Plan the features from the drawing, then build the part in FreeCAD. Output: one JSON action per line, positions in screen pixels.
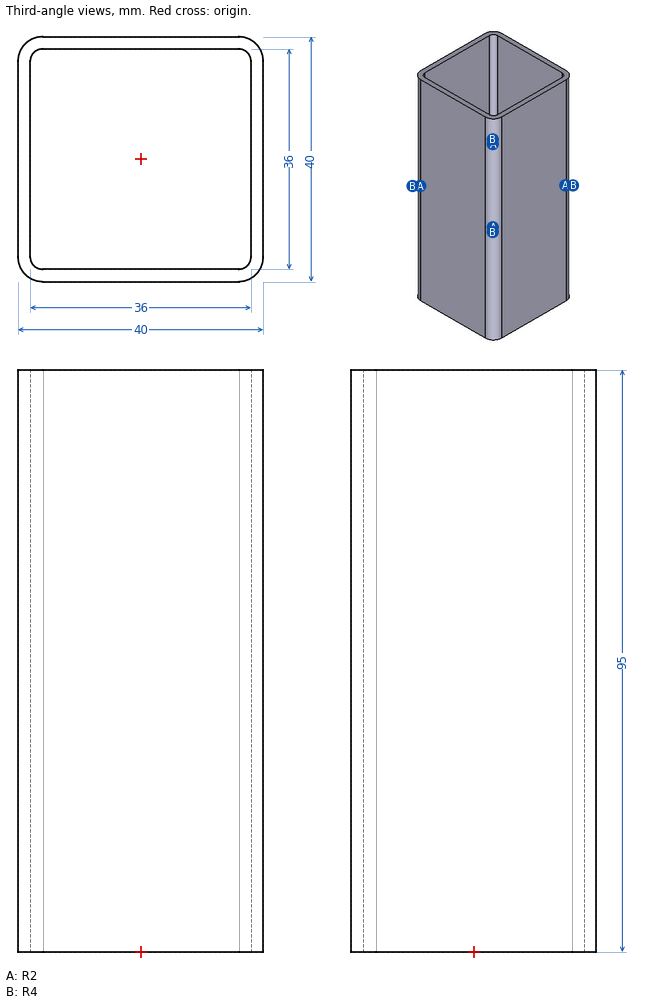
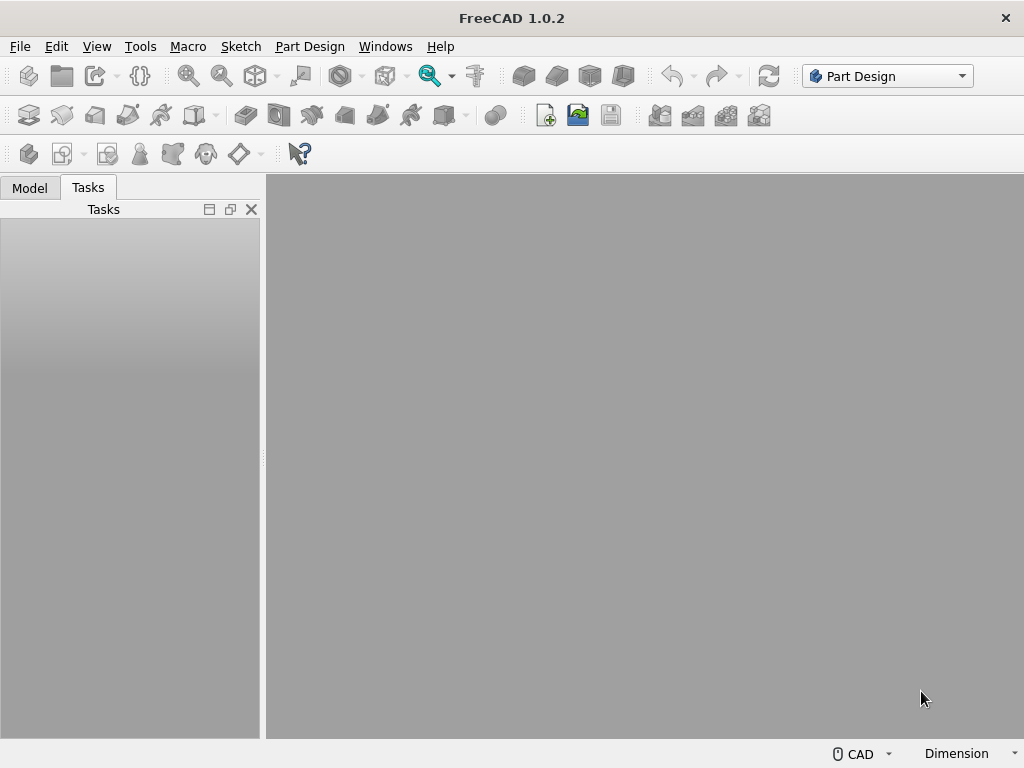
{"action": "left_click", "coordinate": [545, 116]}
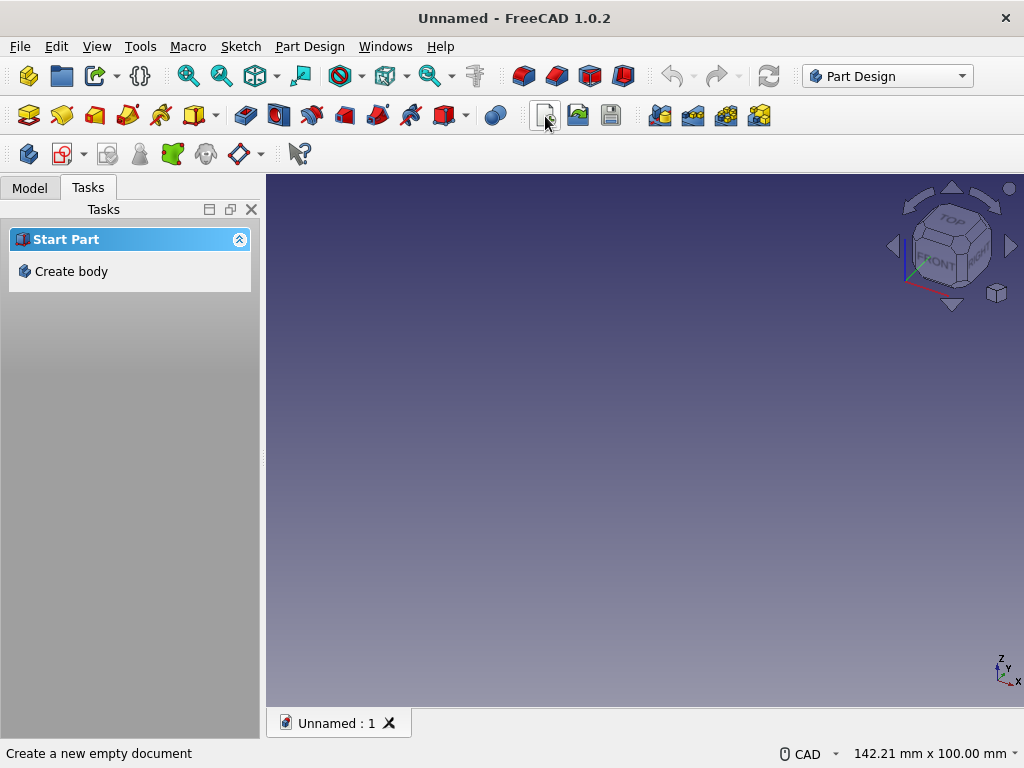
{"action": "left_click", "coordinate": [62, 154]}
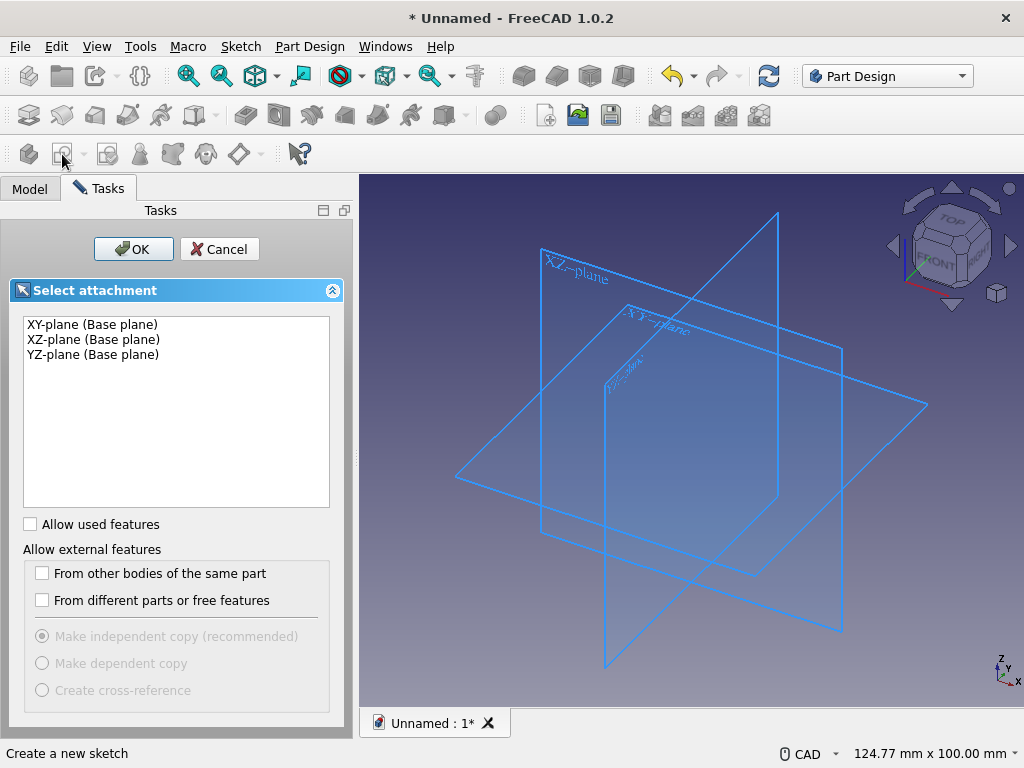
{"action": "left_click", "coordinate": [84, 324]}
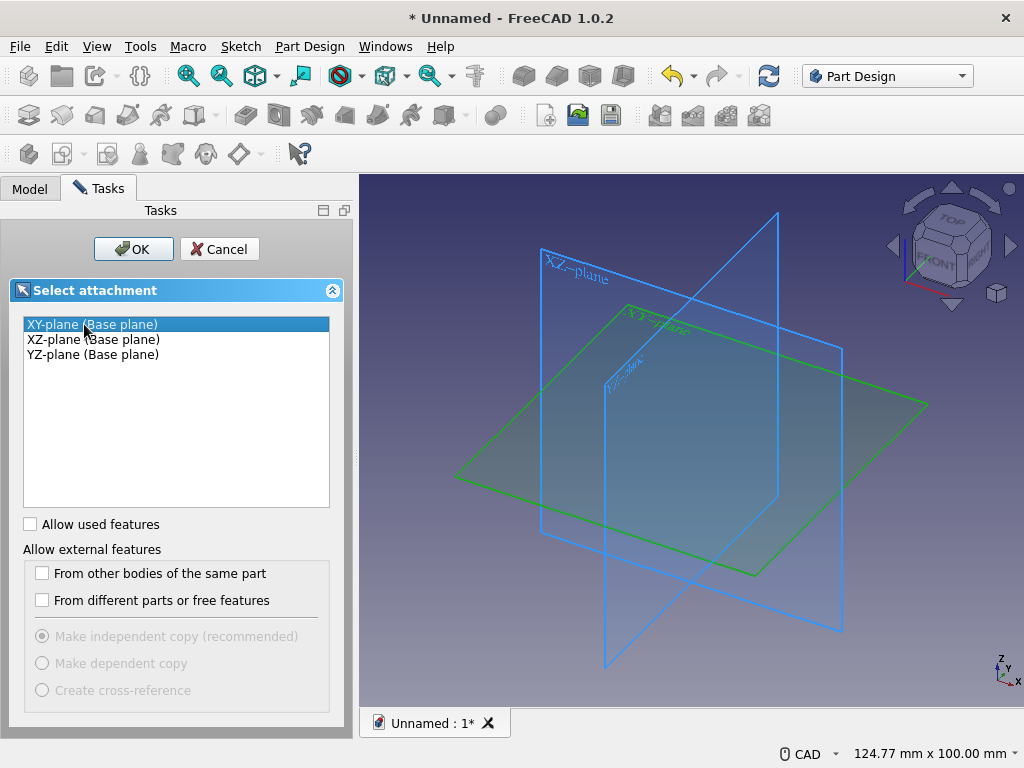
{"action": "left_click", "coordinate": [134, 249]}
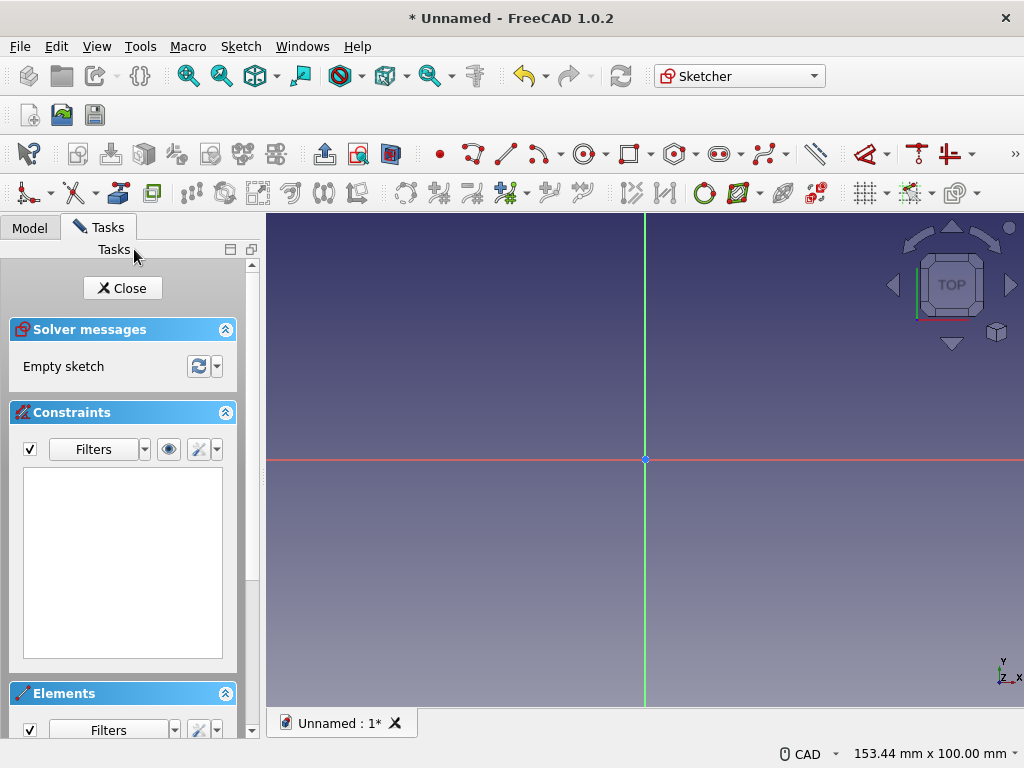
{"action": "scroll", "coordinate": [784, 460], "scroll_direction": "up", "scroll_amount": 2}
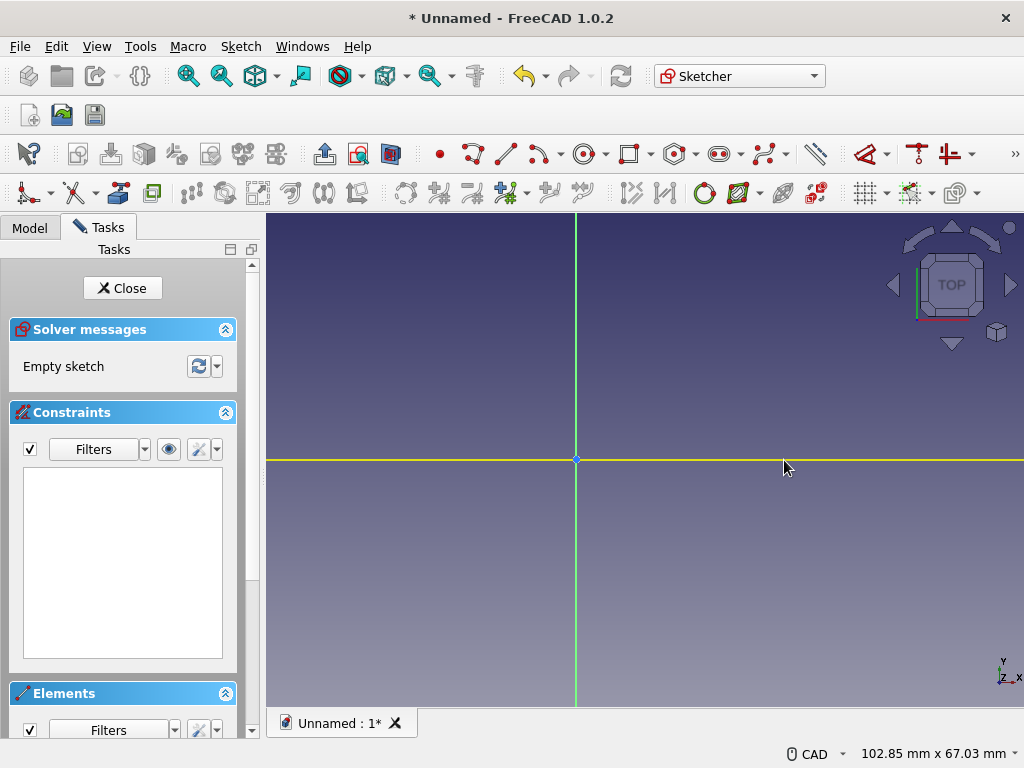
{"action": "key", "text": "g v"}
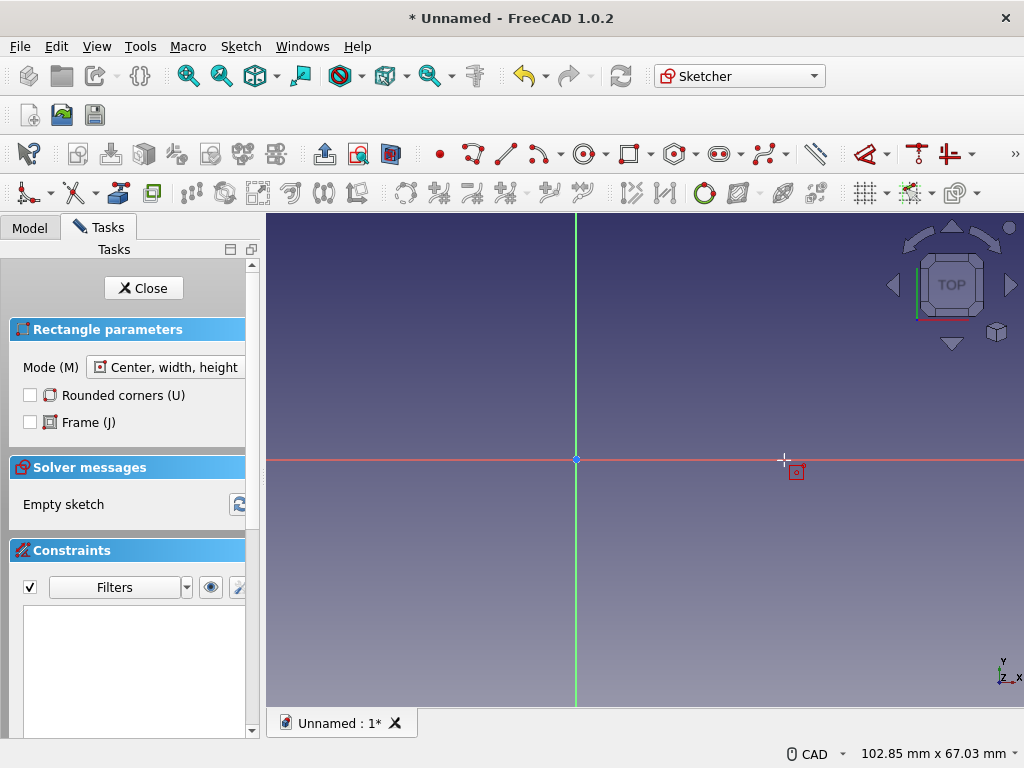
{"action": "left_click", "coordinate": [576, 460]}
{"action": "left_click", "coordinate": [724, 312]}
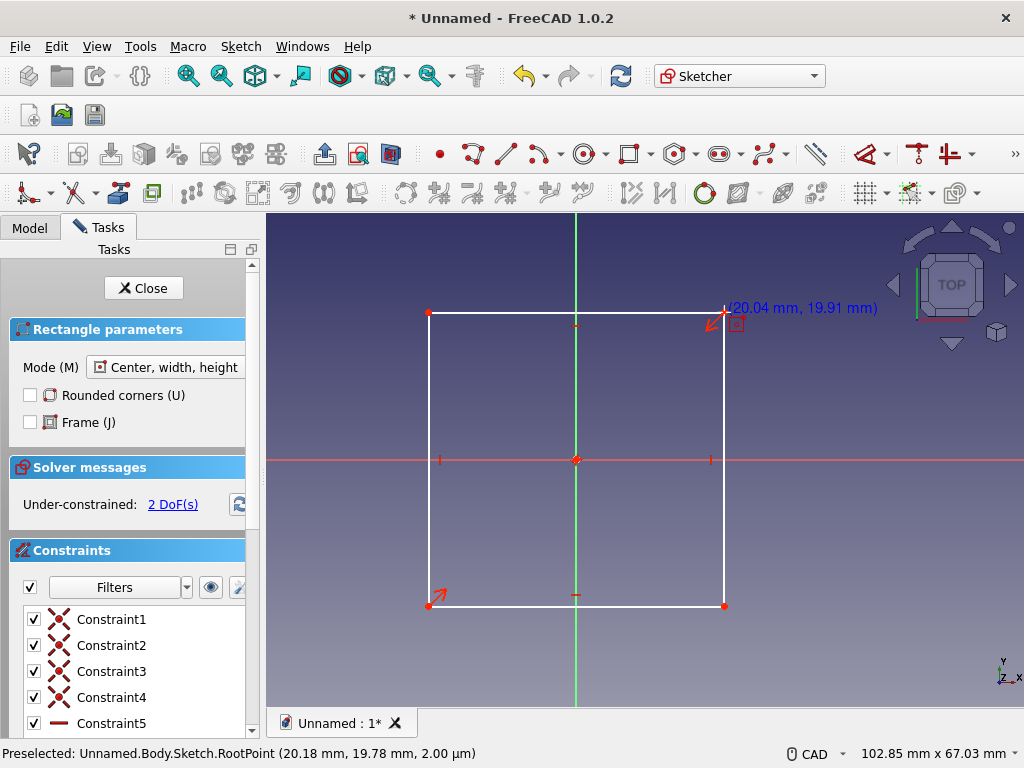
{"action": "left_click", "coordinate": [576, 460]}
{"action": "left_click", "coordinate": [709, 327]}
{"action": "key", "text": "Escape"}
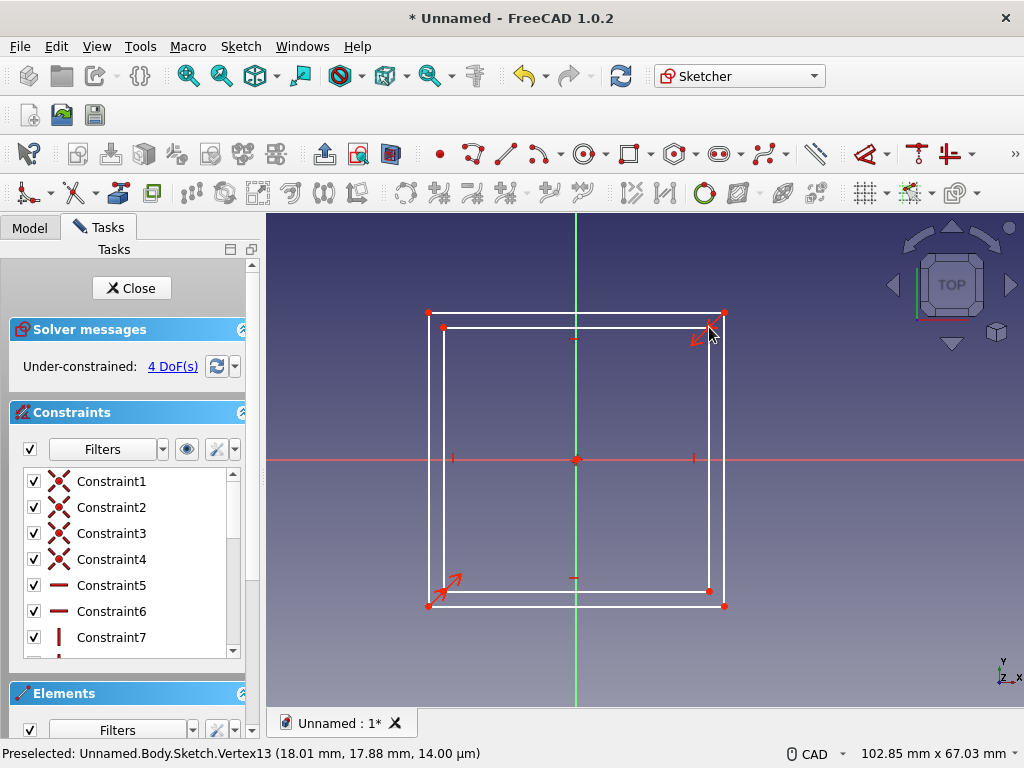
{"action": "left_click", "coordinate": [864, 154]}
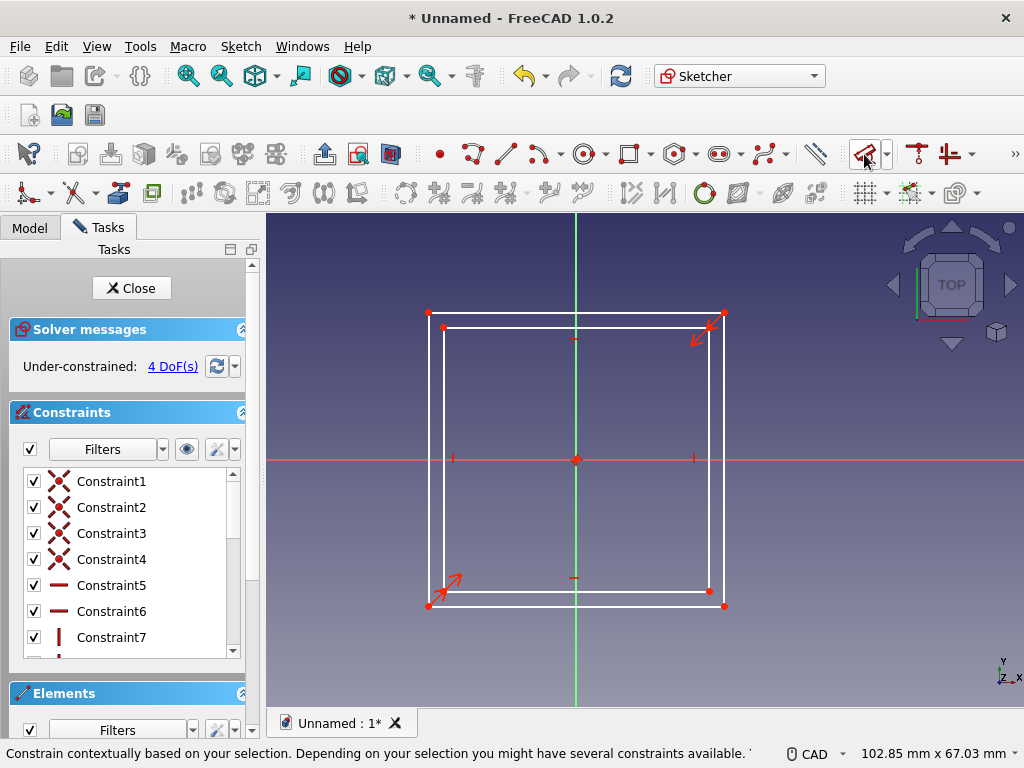
{"action": "left_click", "coordinate": [517, 607]}
{"action": "left_click", "coordinate": [508, 641]}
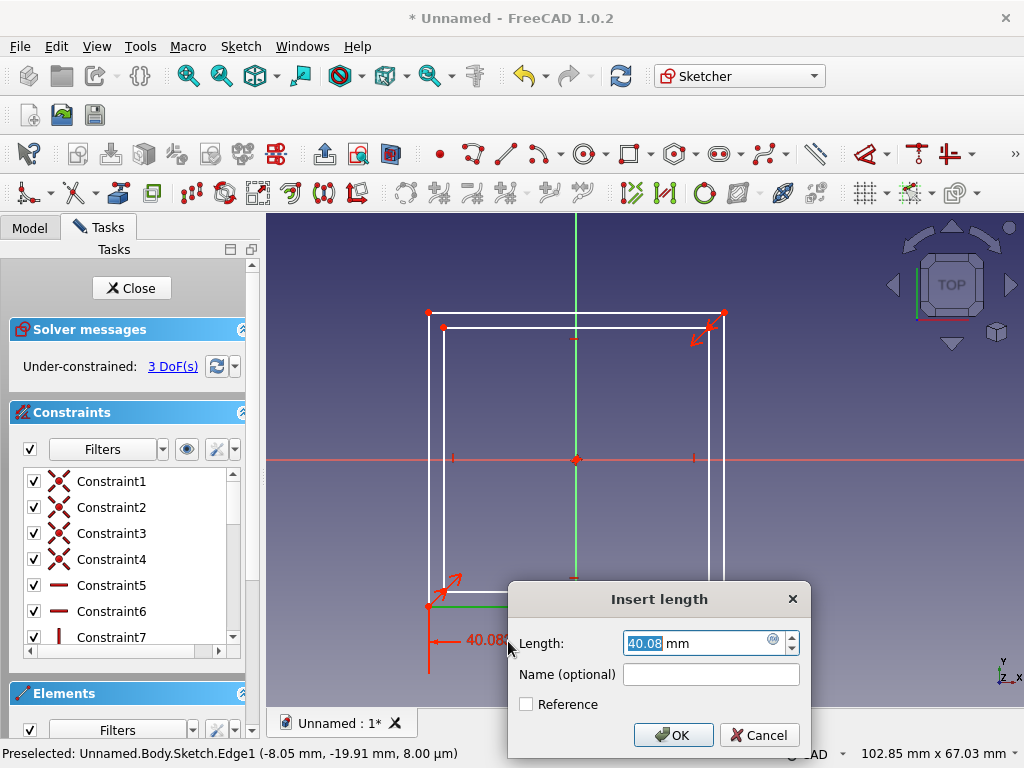
{"action": "type", "text": "40"}
{"action": "key", "text": "Return"}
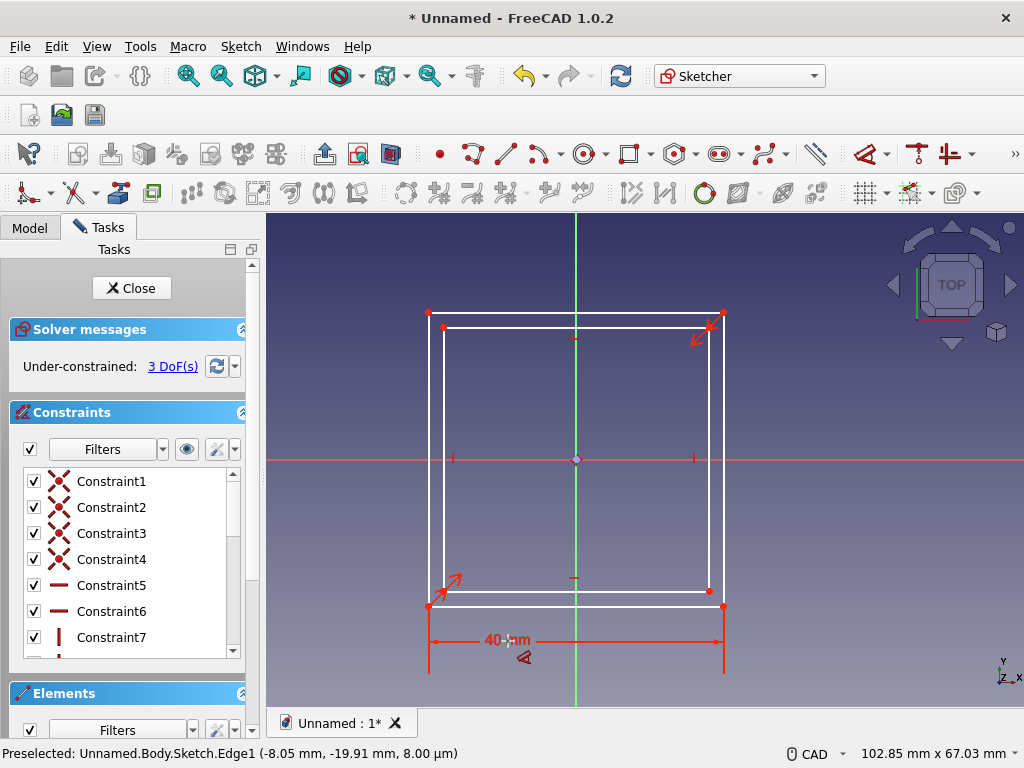
{"action": "left_click", "coordinate": [724, 518]}
{"action": "left_click", "coordinate": [758, 392]}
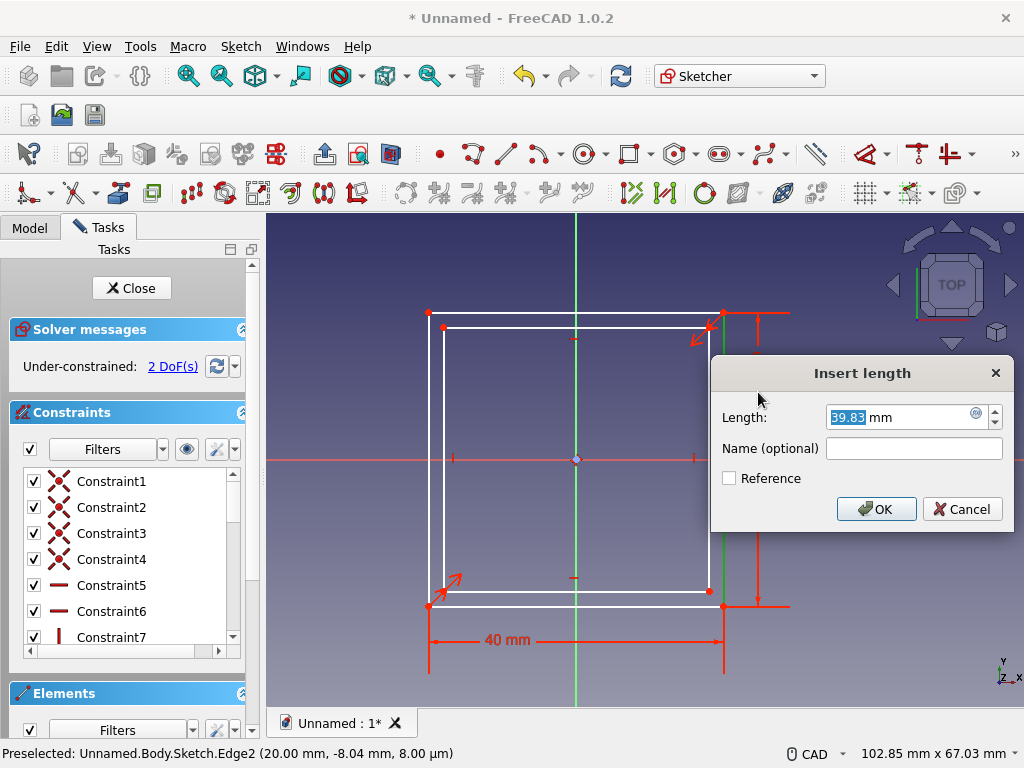
{"action": "type", "text": "40"}
{"action": "key", "text": "Return"}